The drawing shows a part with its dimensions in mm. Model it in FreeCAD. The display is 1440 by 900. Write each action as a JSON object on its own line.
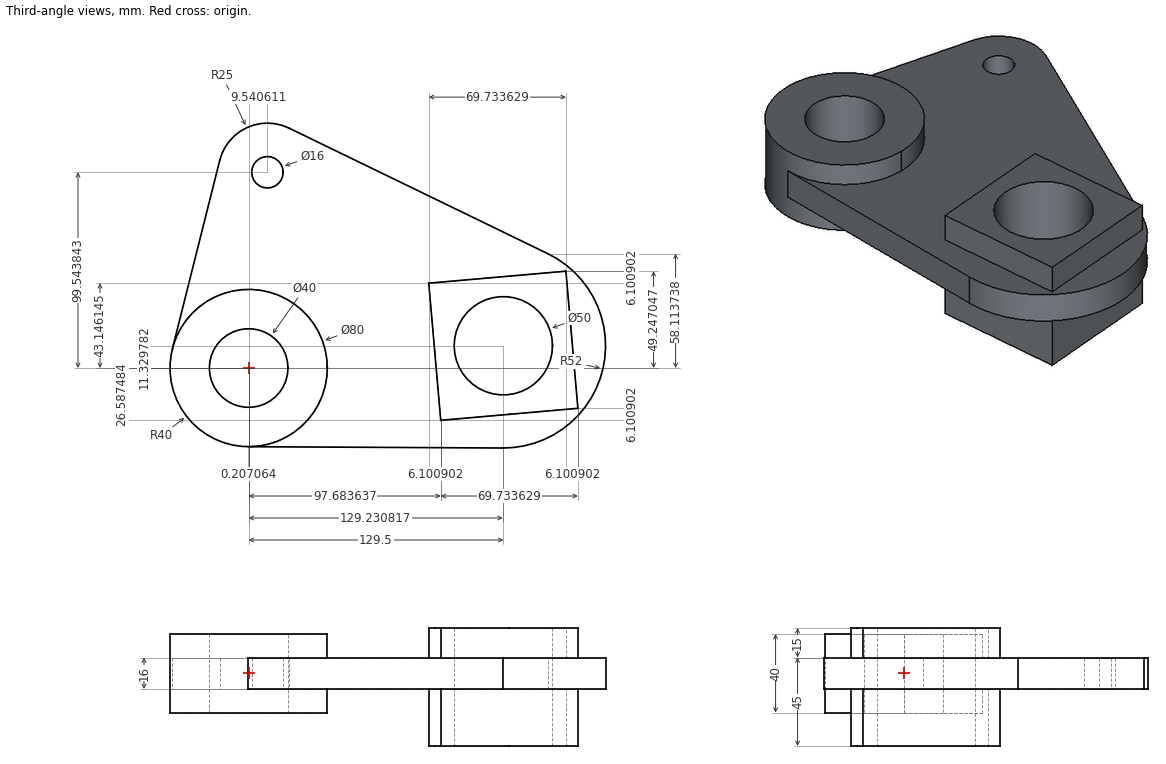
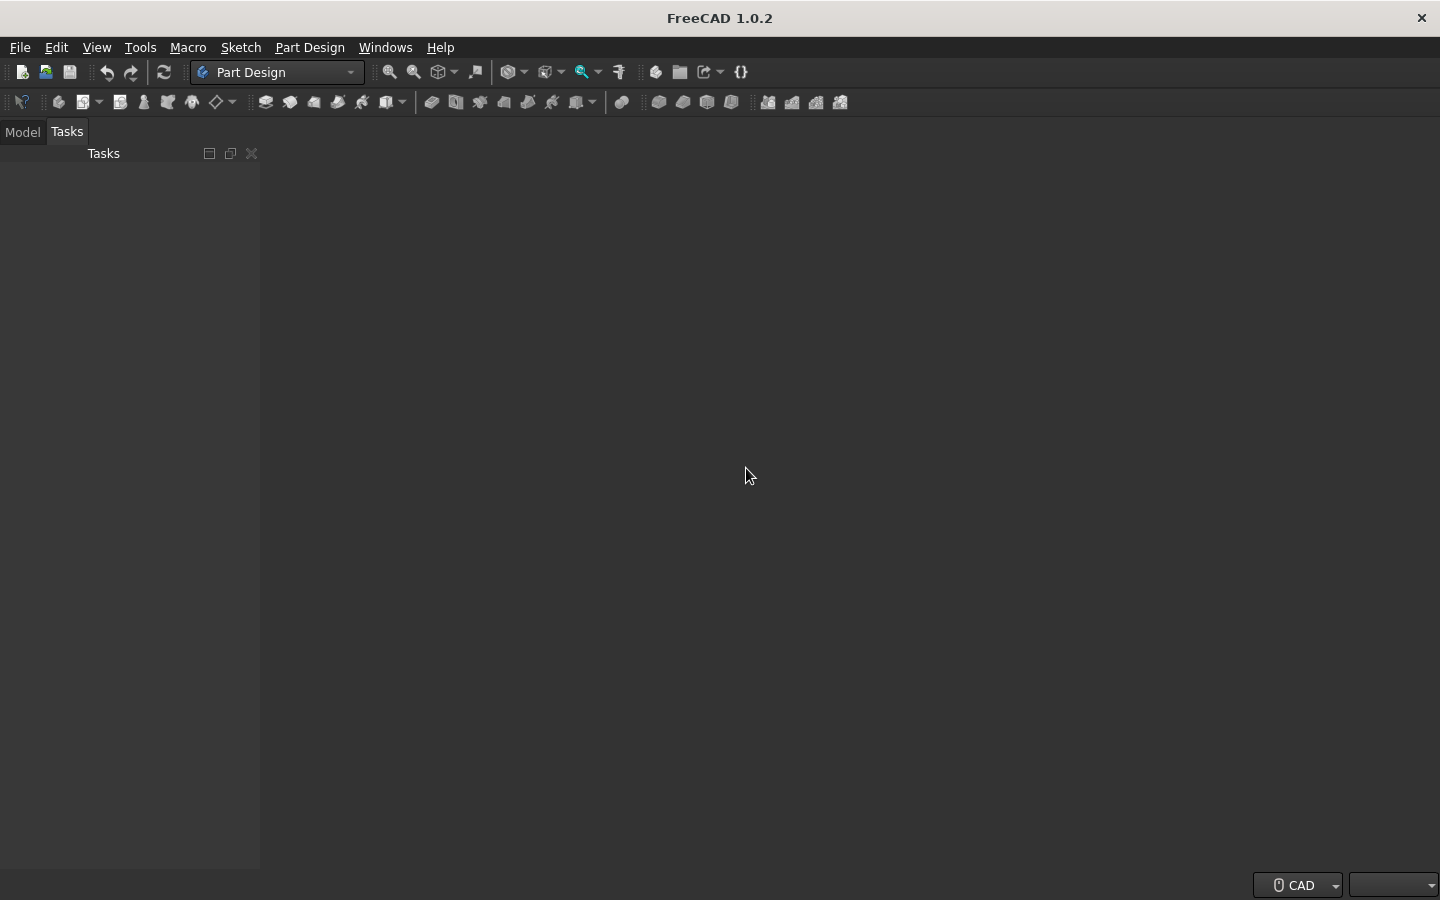
{"action": "left_click", "coordinate": [22, 72]}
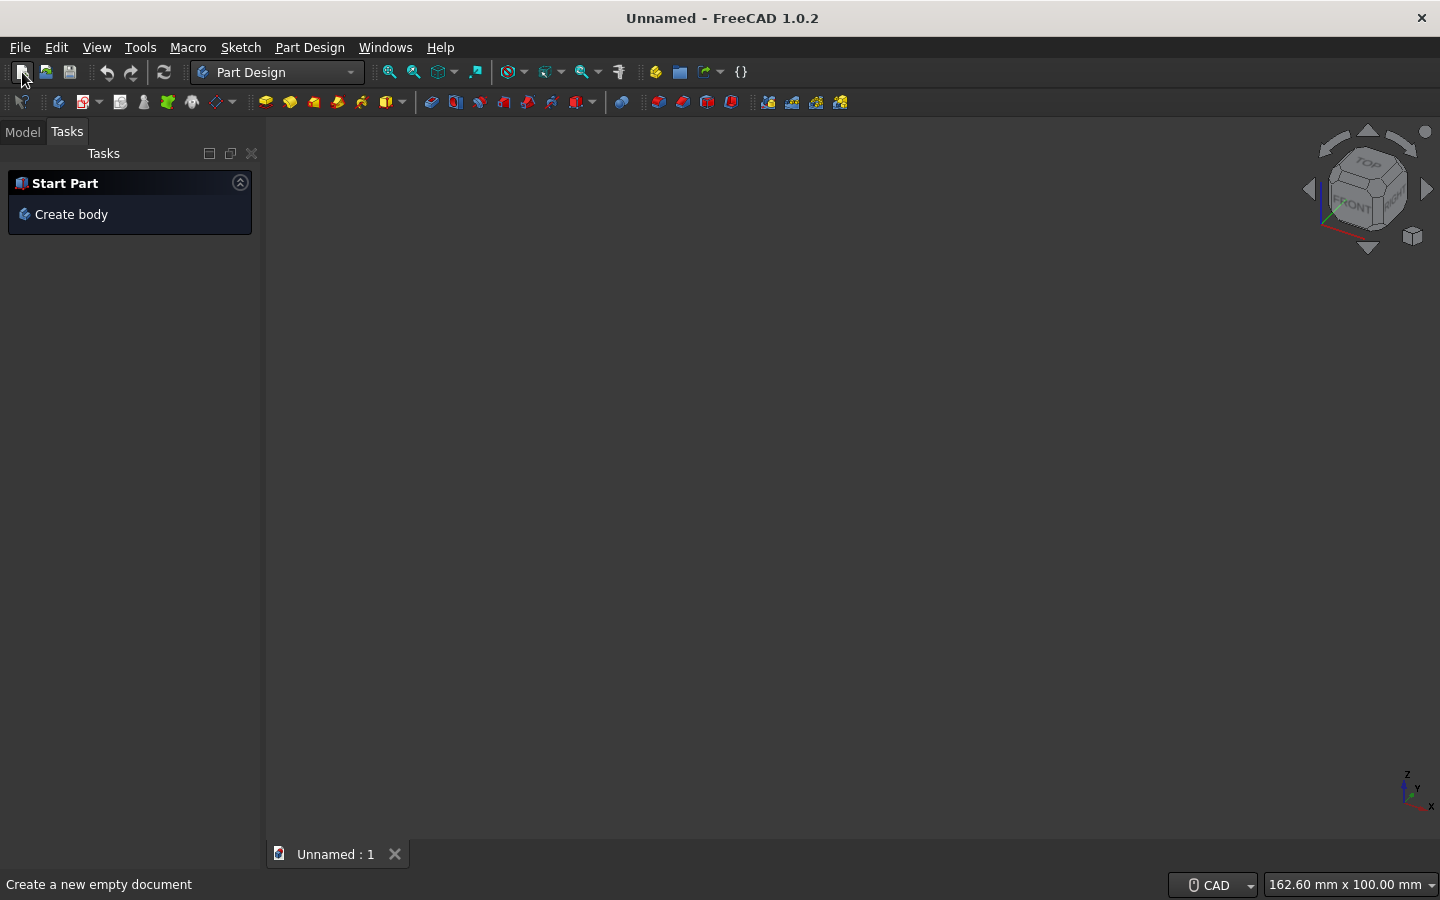
{"action": "left_click", "coordinate": [84, 102]}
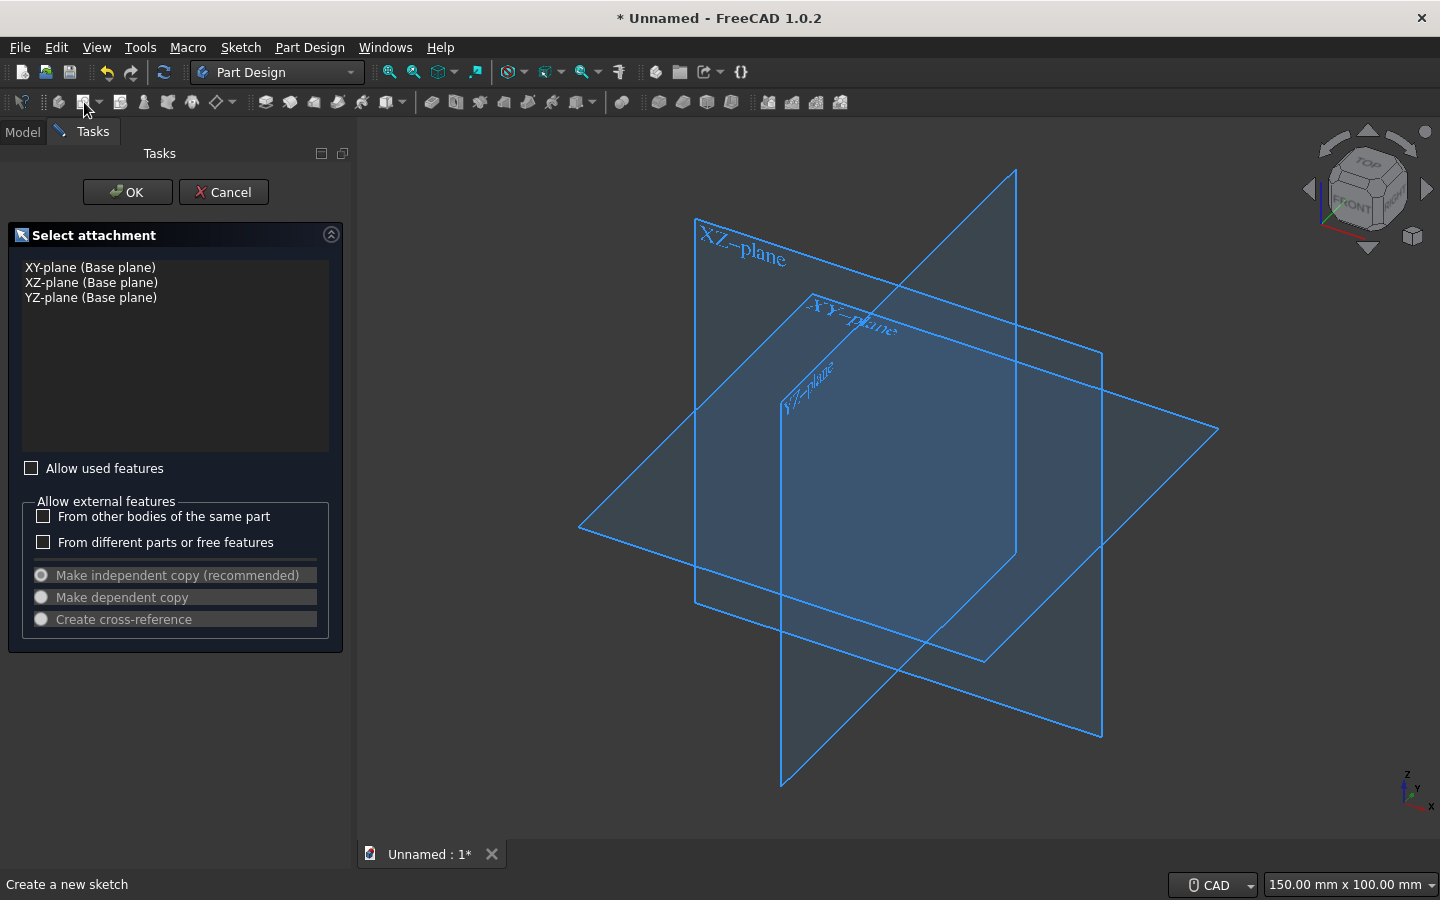
{"action": "left_click", "coordinate": [82, 268]}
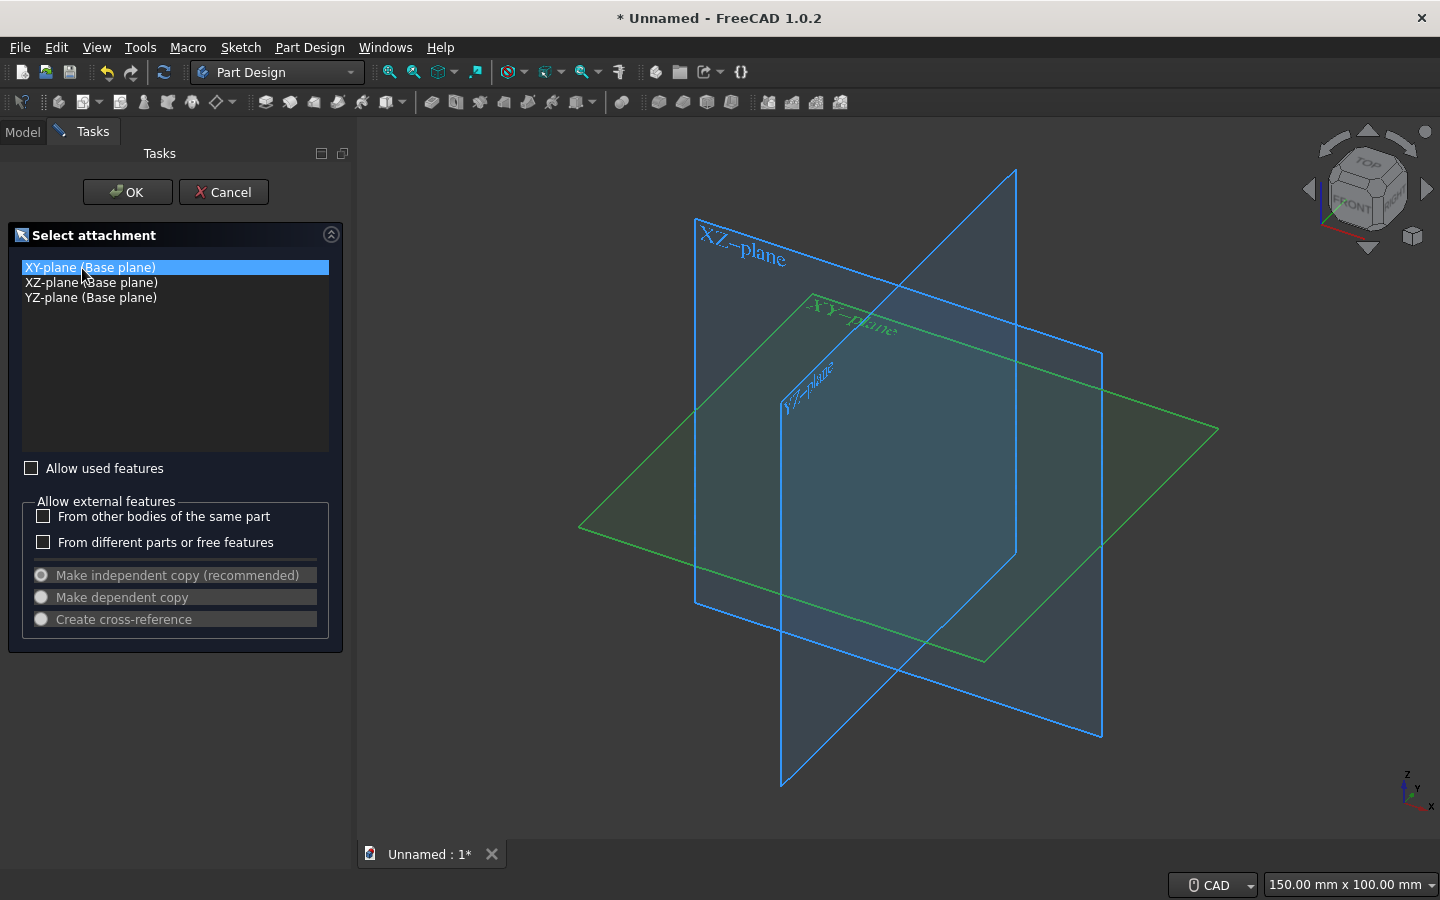
{"action": "left_click", "coordinate": [128, 192]}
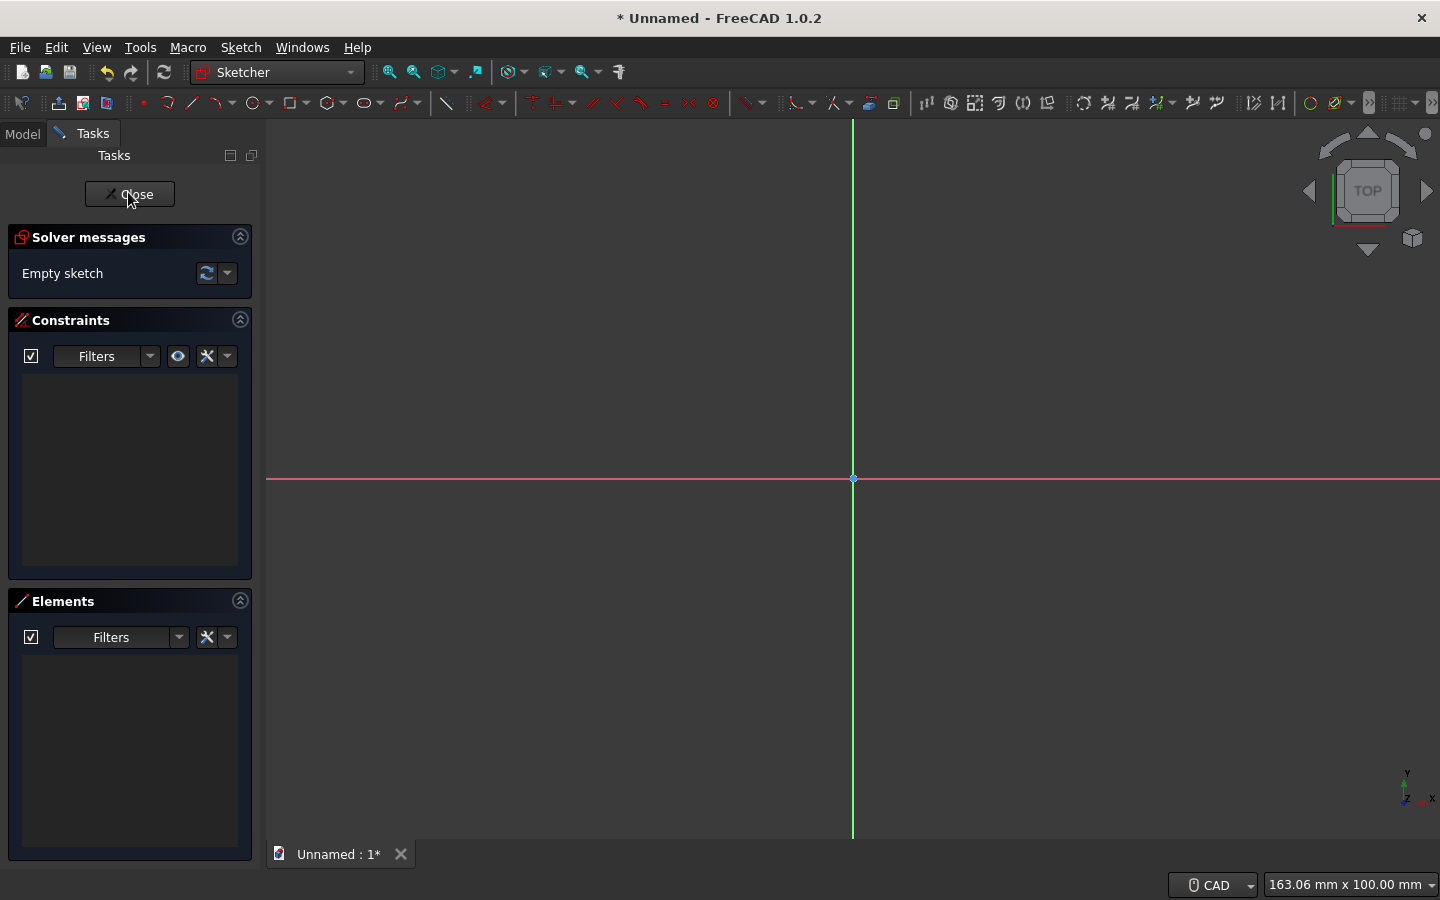
{"action": "left_click", "coordinate": [254, 104]}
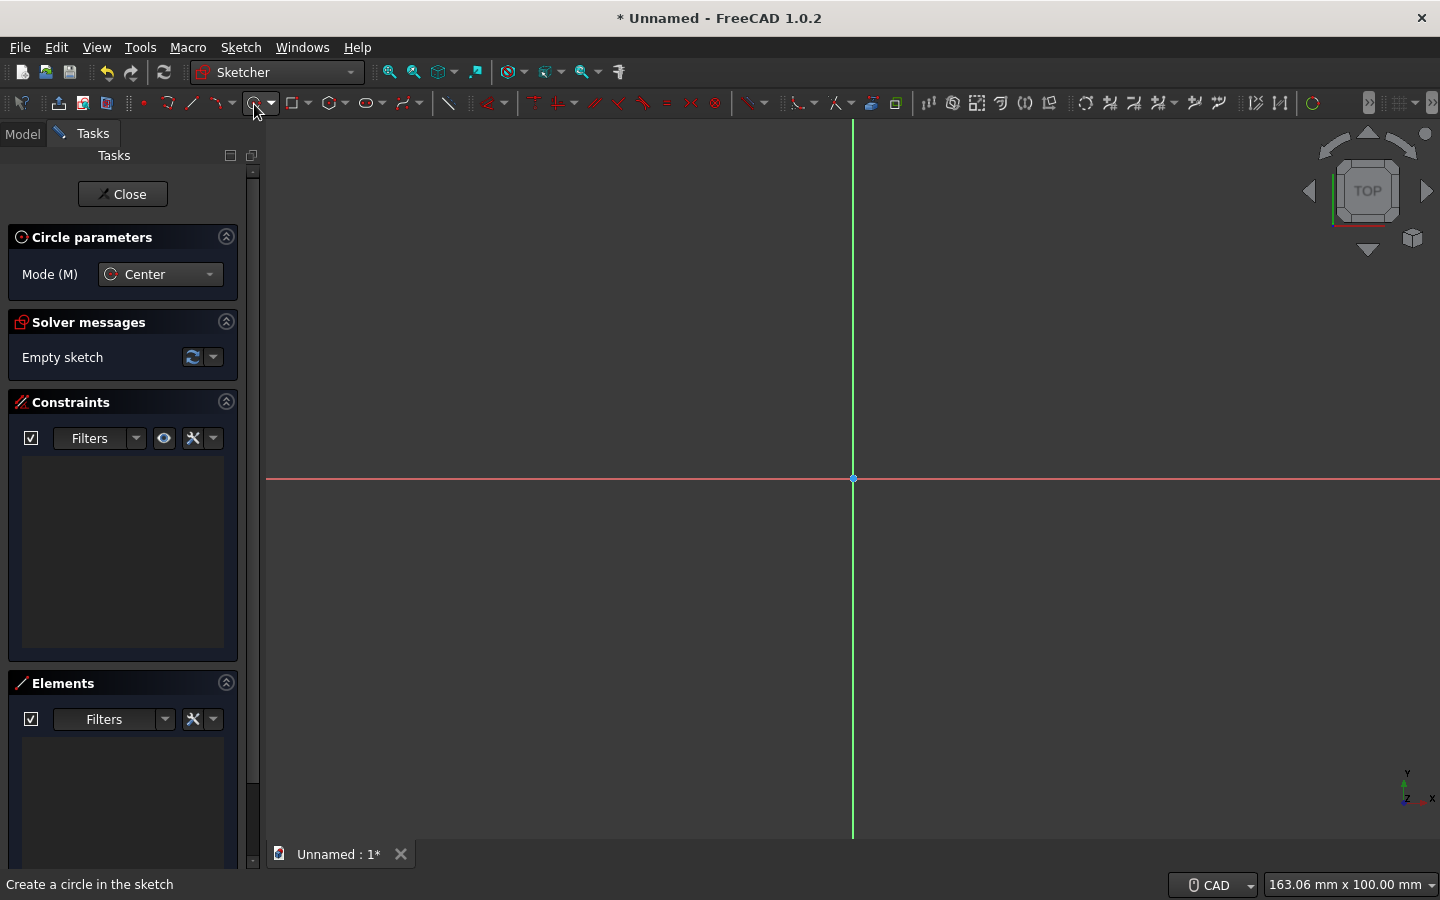
{"action": "left_click", "coordinate": [853, 479]}
{"action": "left_click", "coordinate": [1057, 275]}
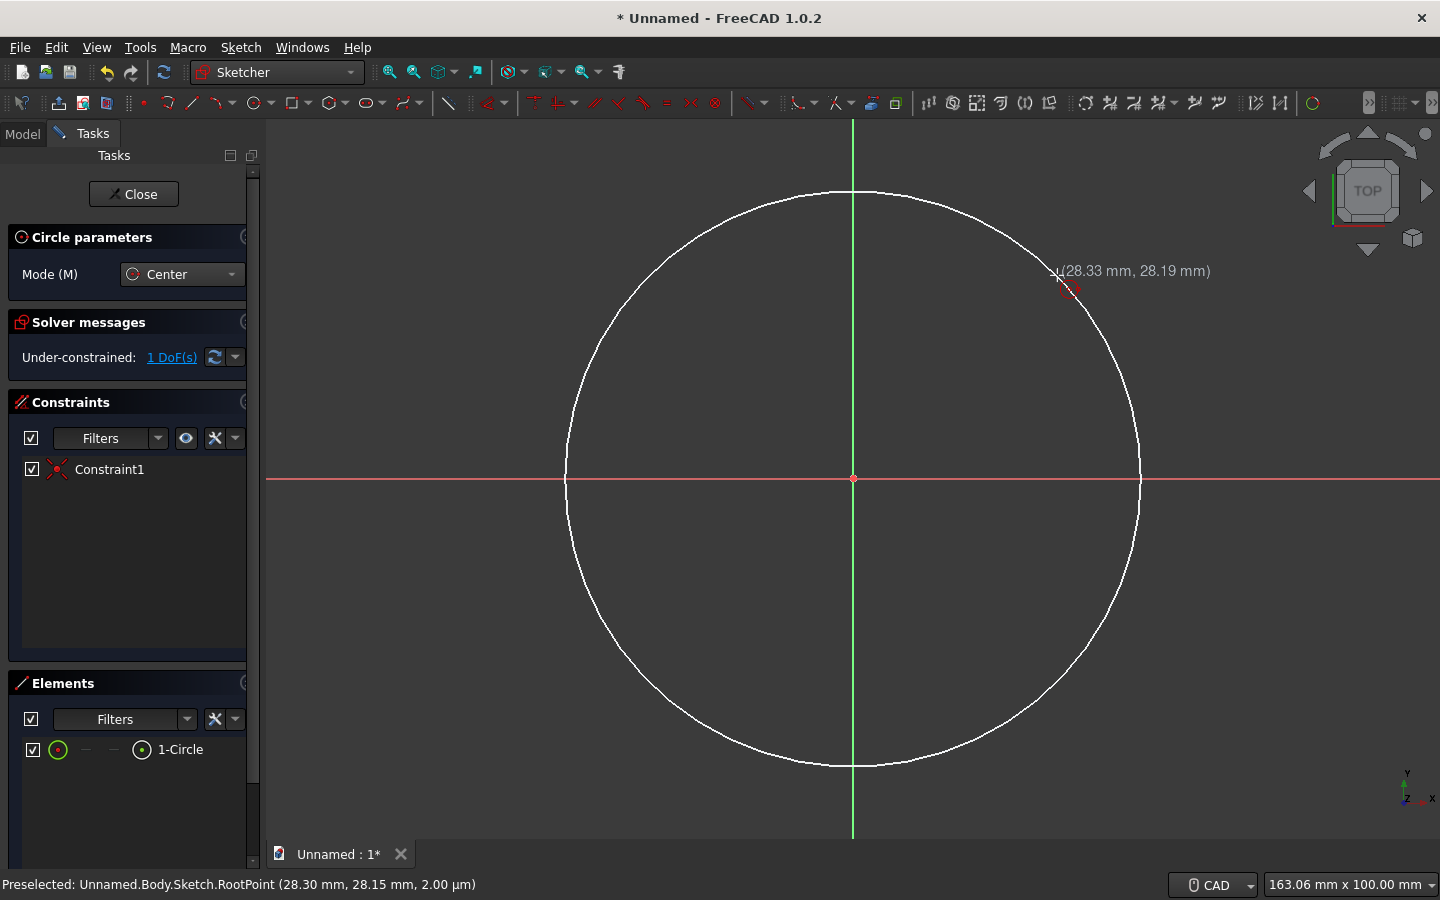
{"action": "left_click", "coordinate": [853, 479]}
{"action": "left_click", "coordinate": [955, 377]}
{"action": "key", "text": "Escape"}